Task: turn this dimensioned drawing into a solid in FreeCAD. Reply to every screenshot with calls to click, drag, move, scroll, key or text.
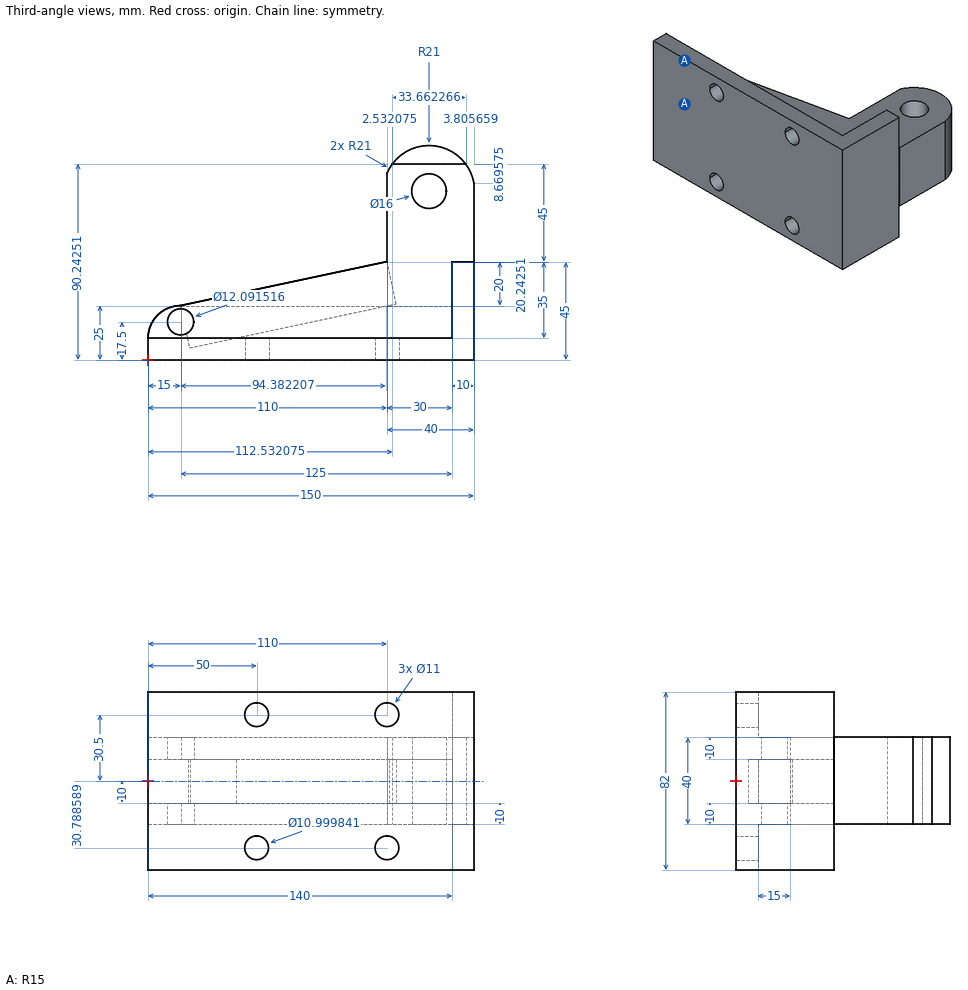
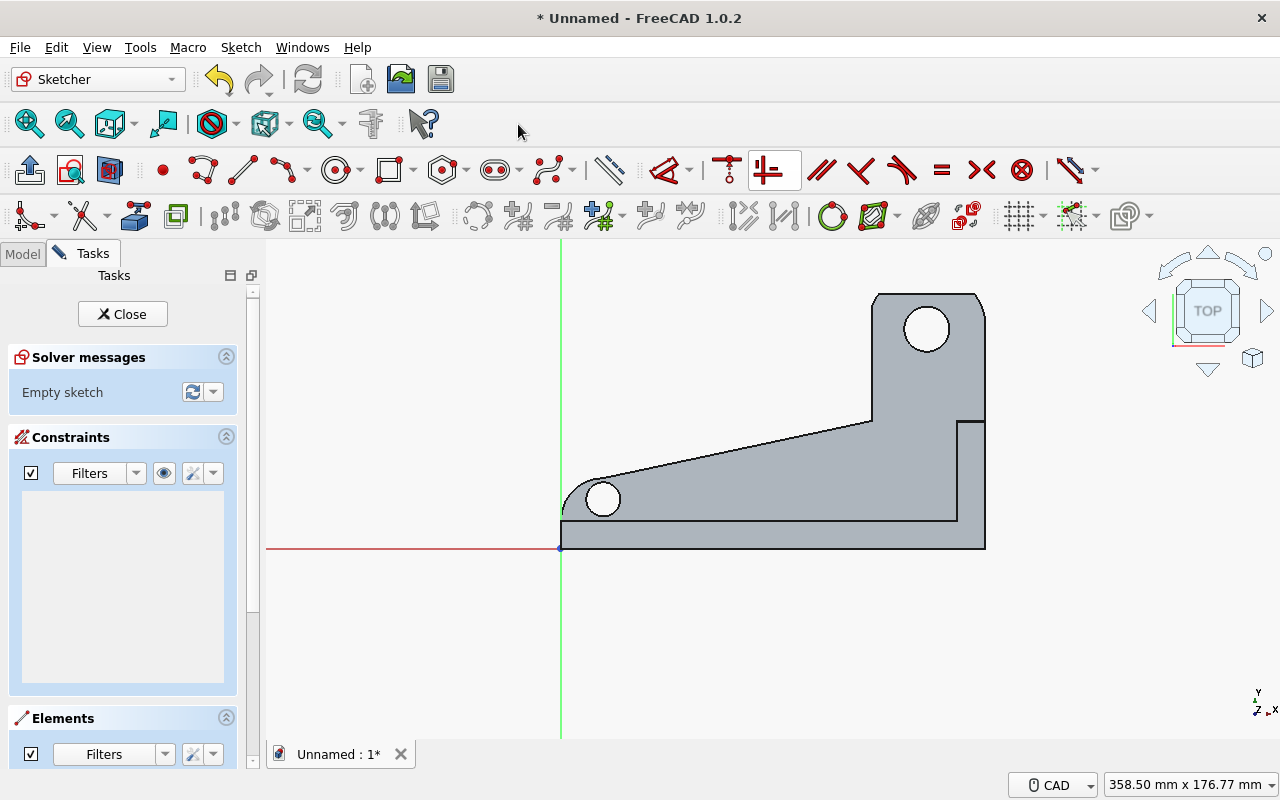
scroll(704, 489, down, 5)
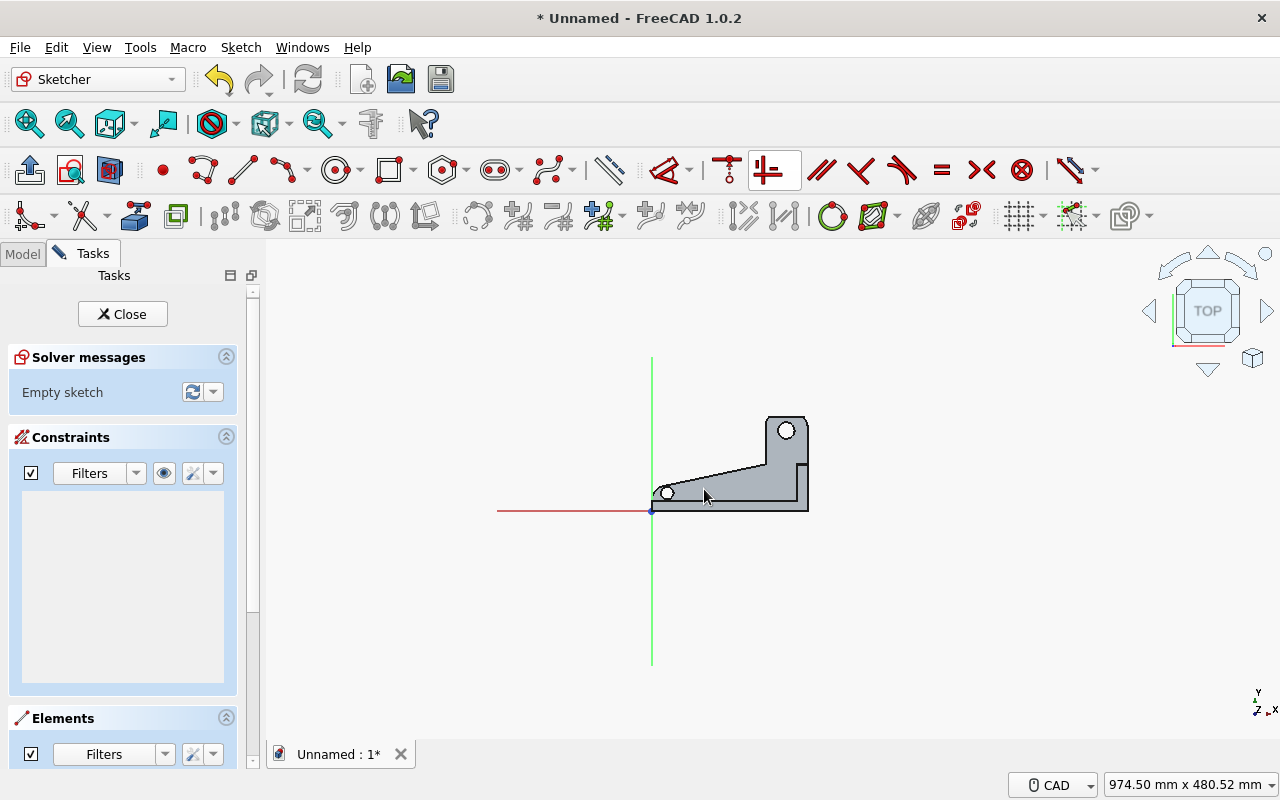
scroll(792, 408, up, 14)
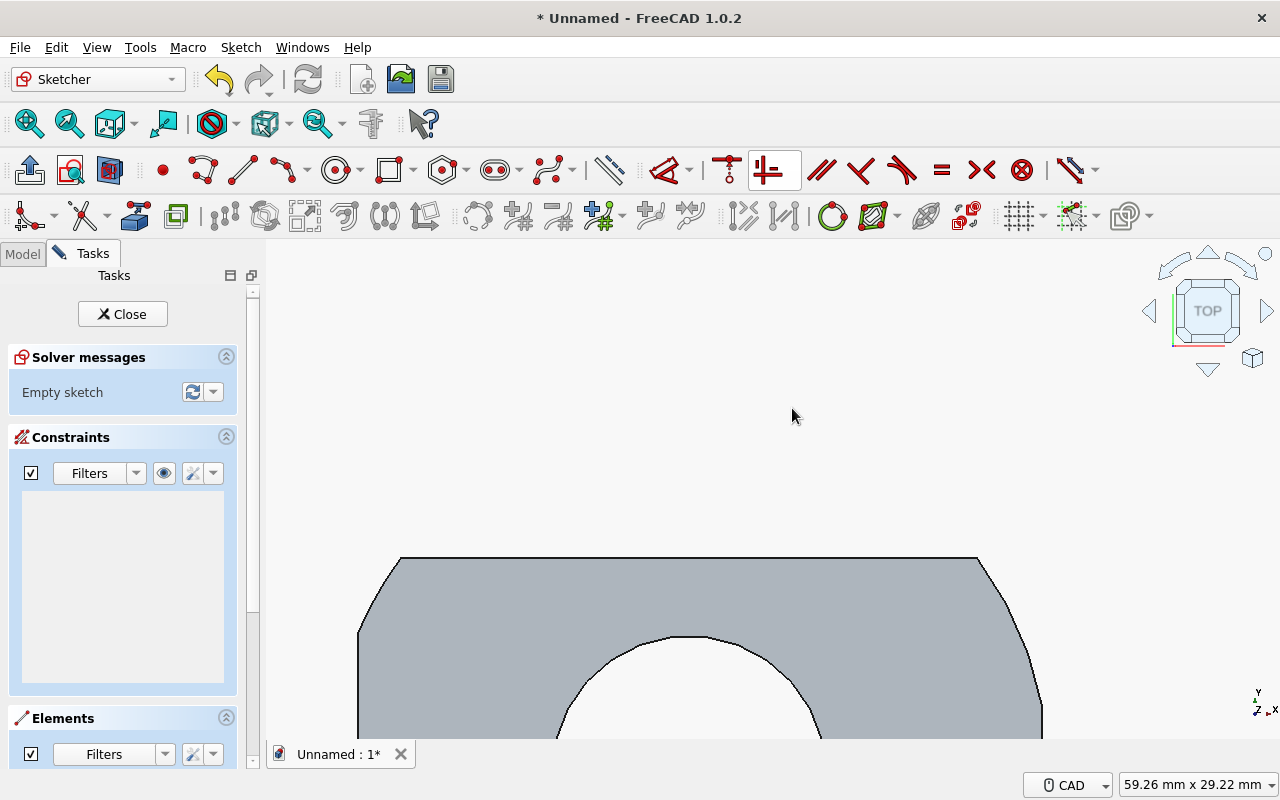
click(244, 170)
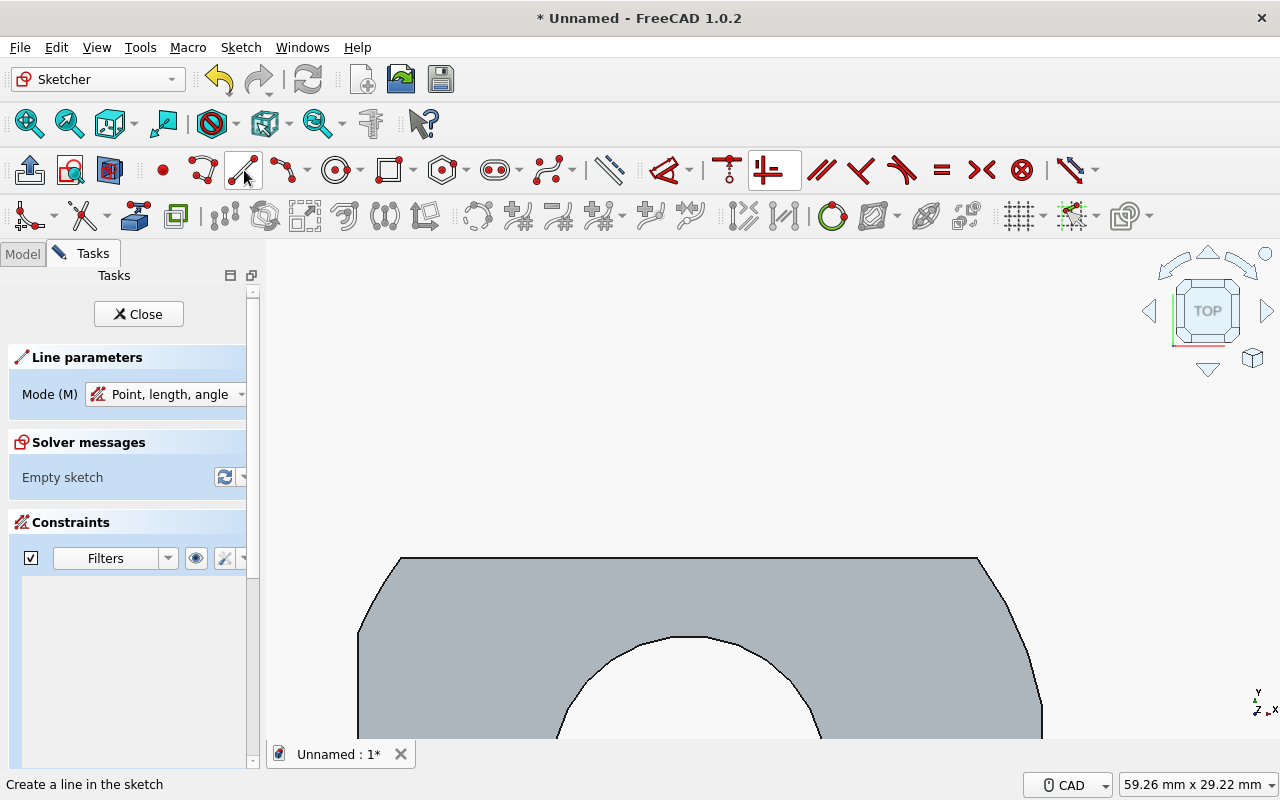
click(401, 558)
click(977, 558)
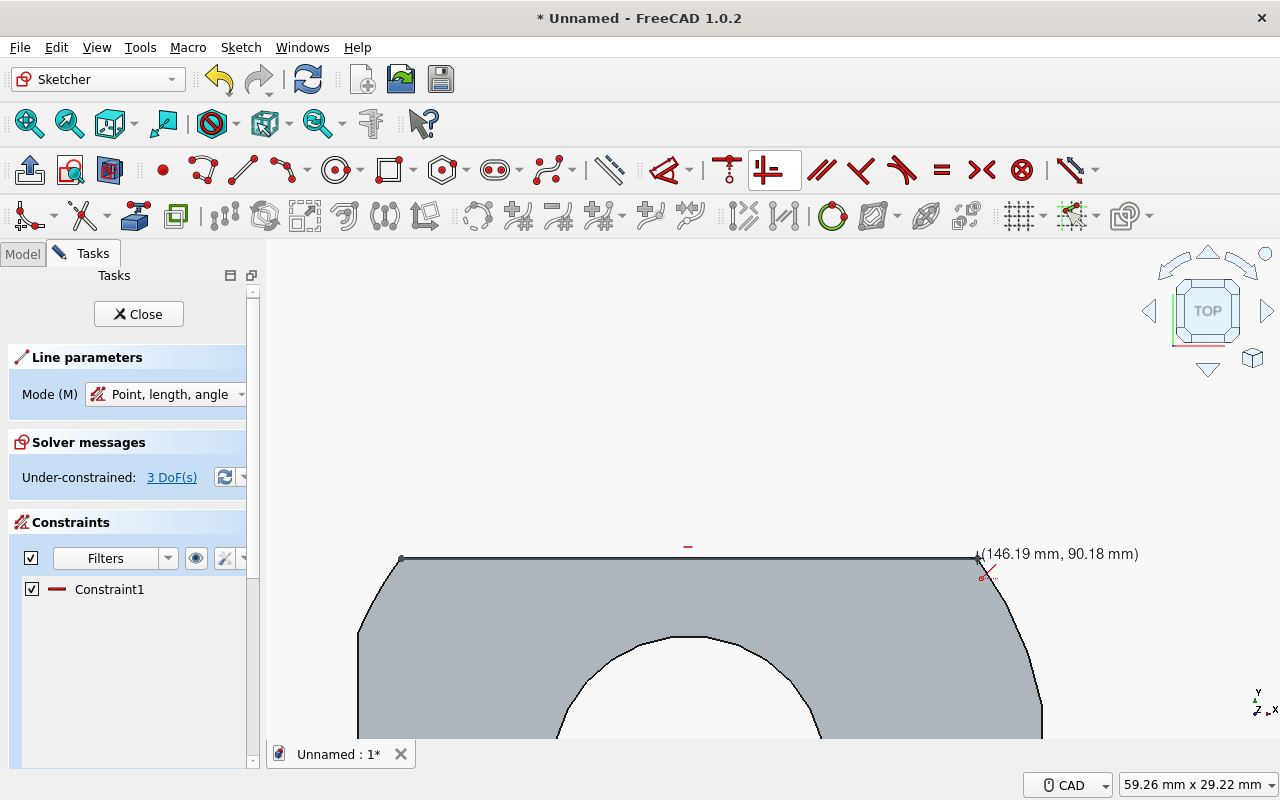
click(284, 170)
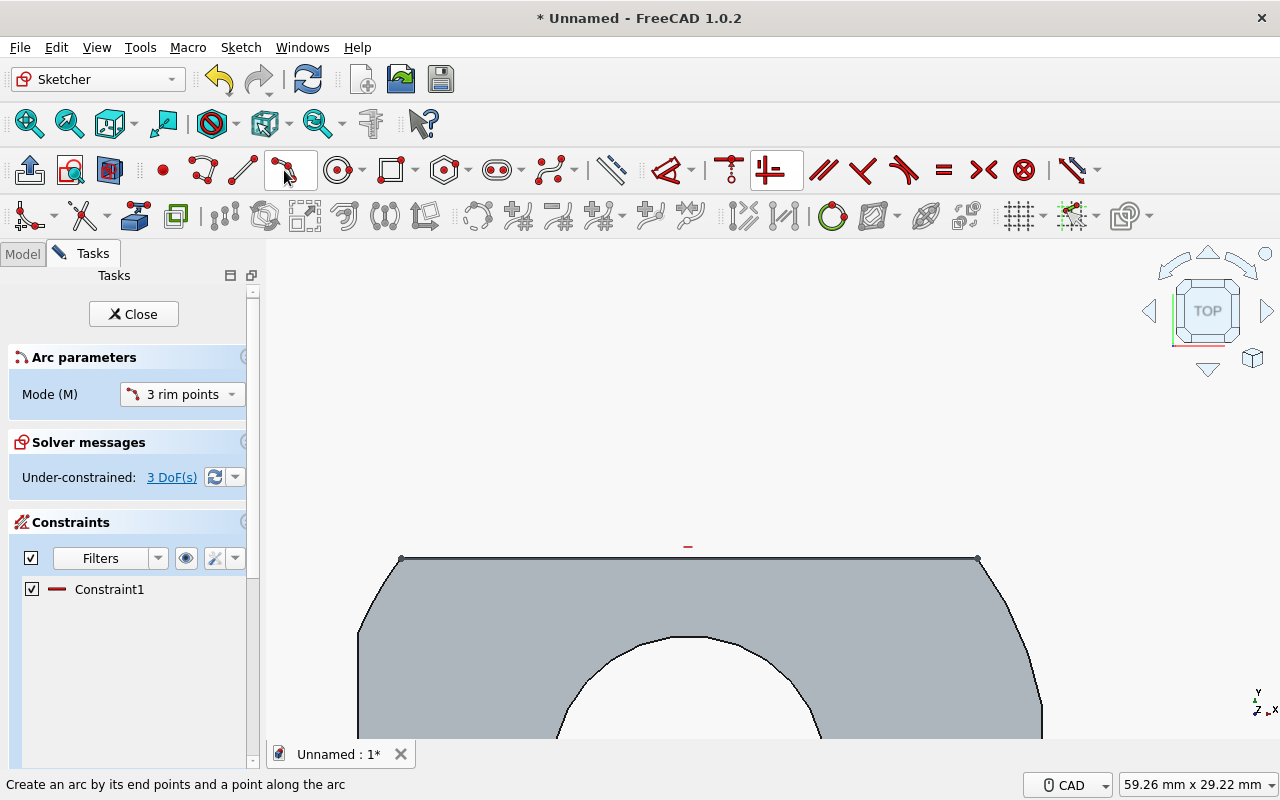
click(977, 559)
click(401, 559)
click(689, 414)
key(Escape)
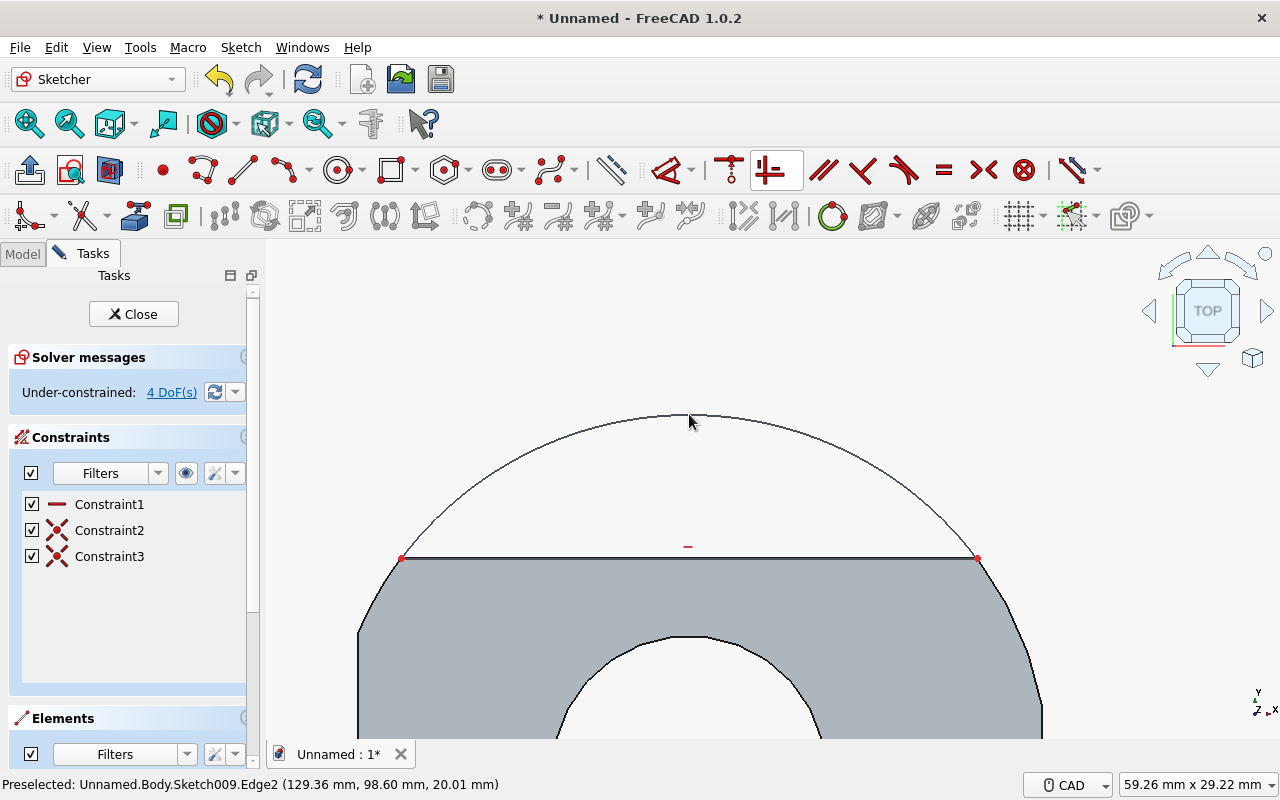
click(666, 170)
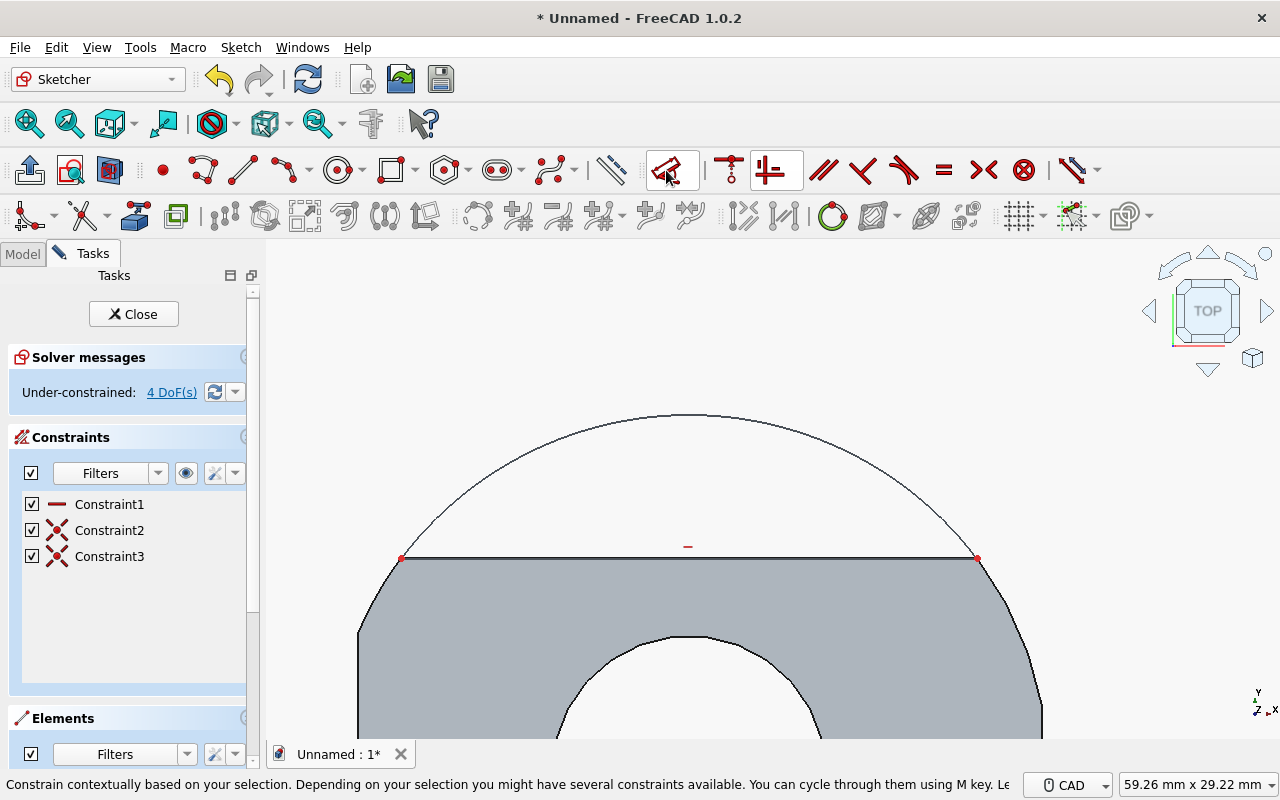
click(819, 439)
click(831, 409)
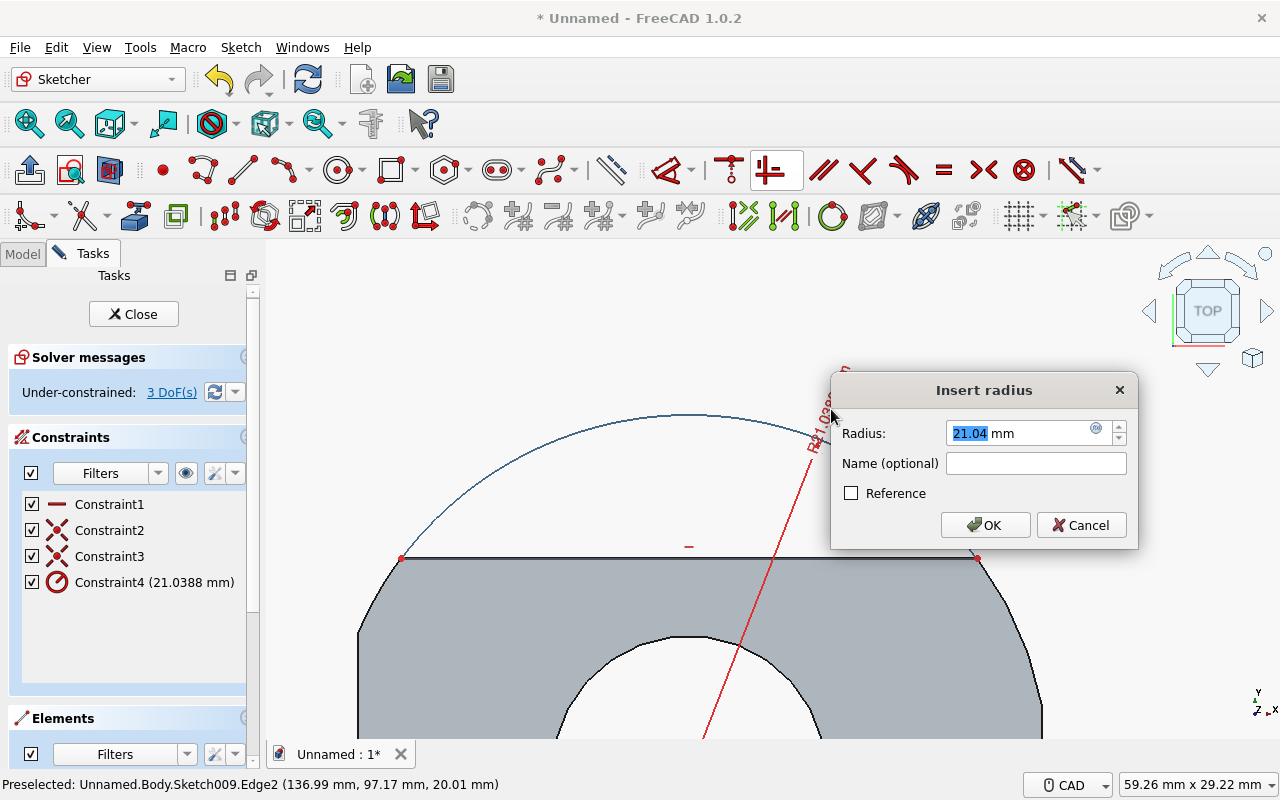
text(21)
key(Return)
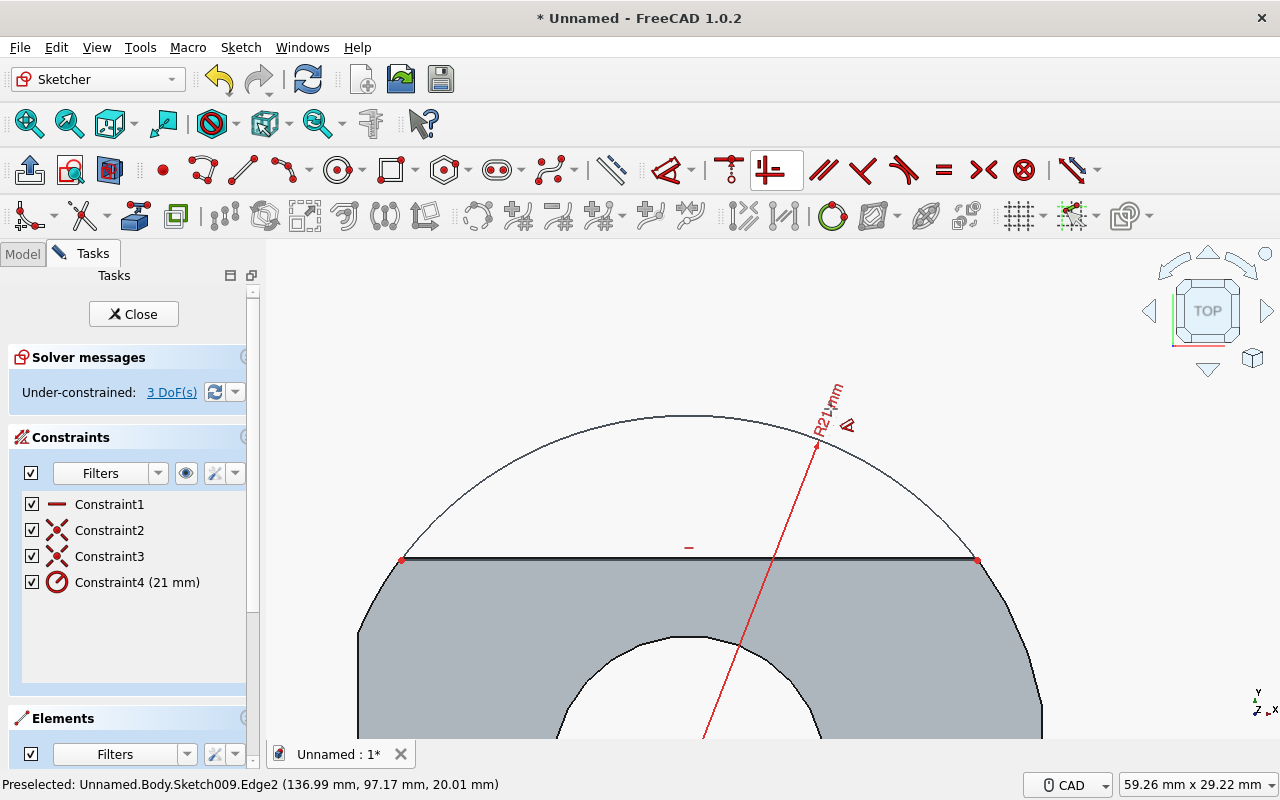
click(574, 560)
click(689, 594)